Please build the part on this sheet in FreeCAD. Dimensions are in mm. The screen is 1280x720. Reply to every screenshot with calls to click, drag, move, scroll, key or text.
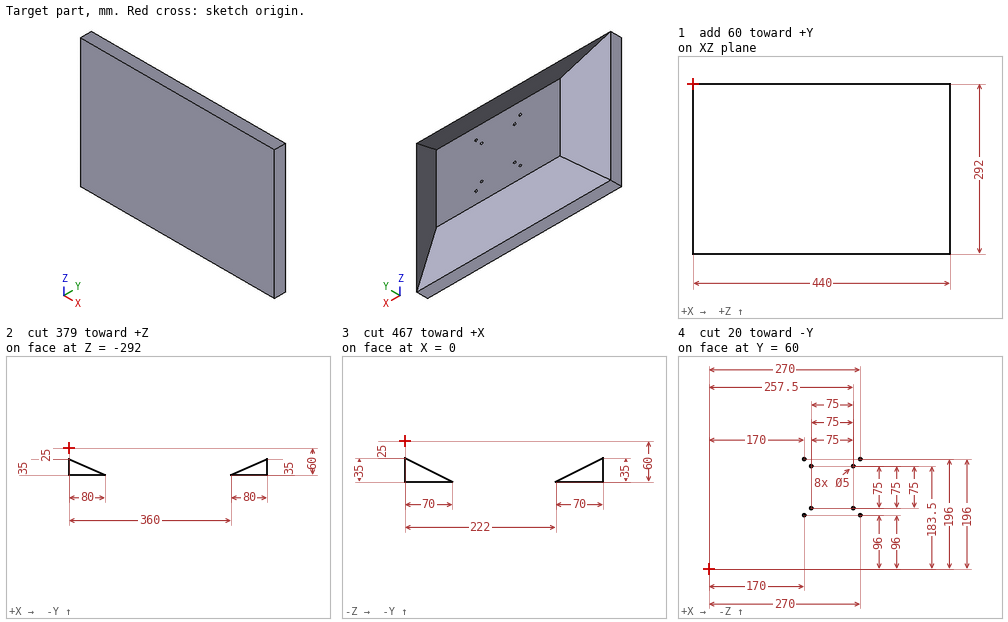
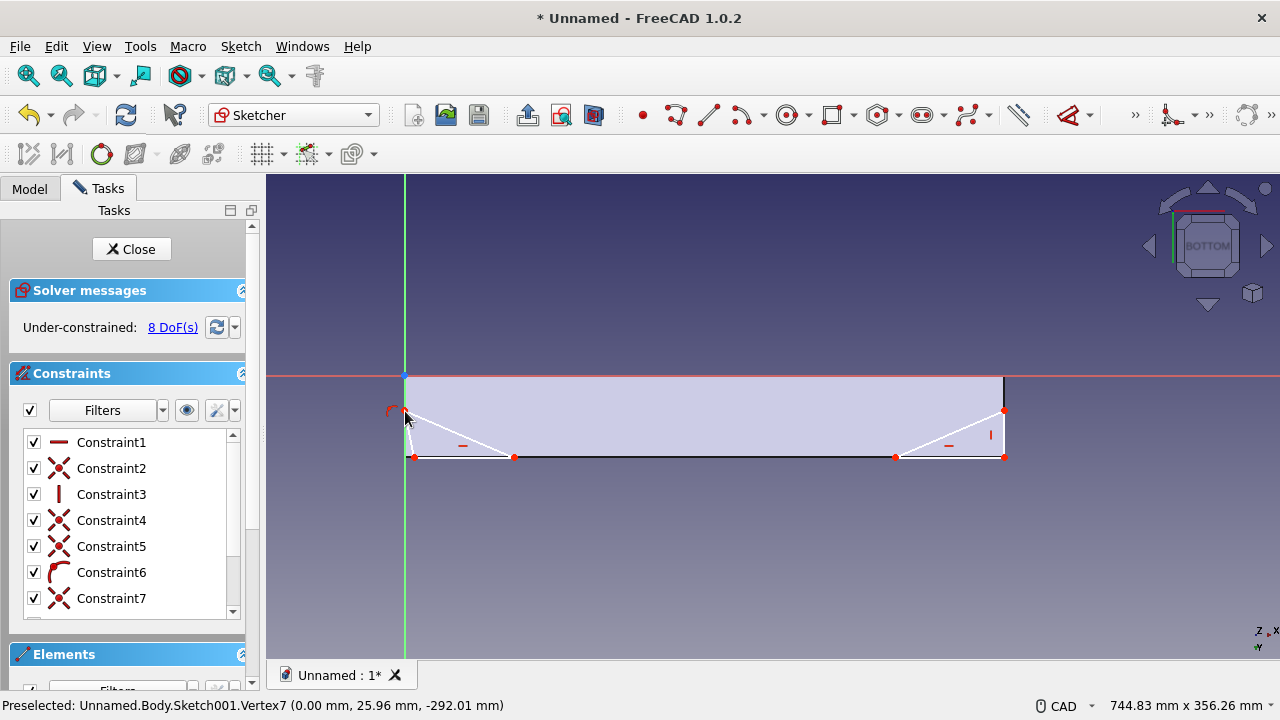
click(408, 425)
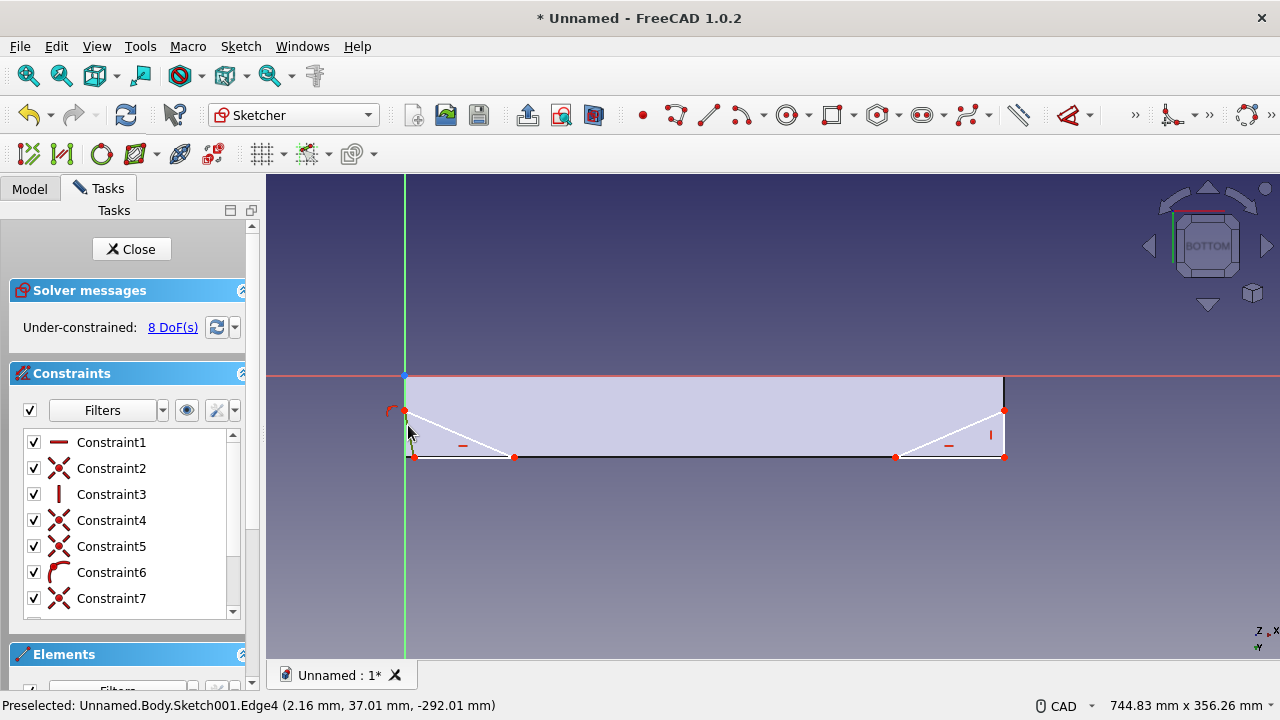
key(v)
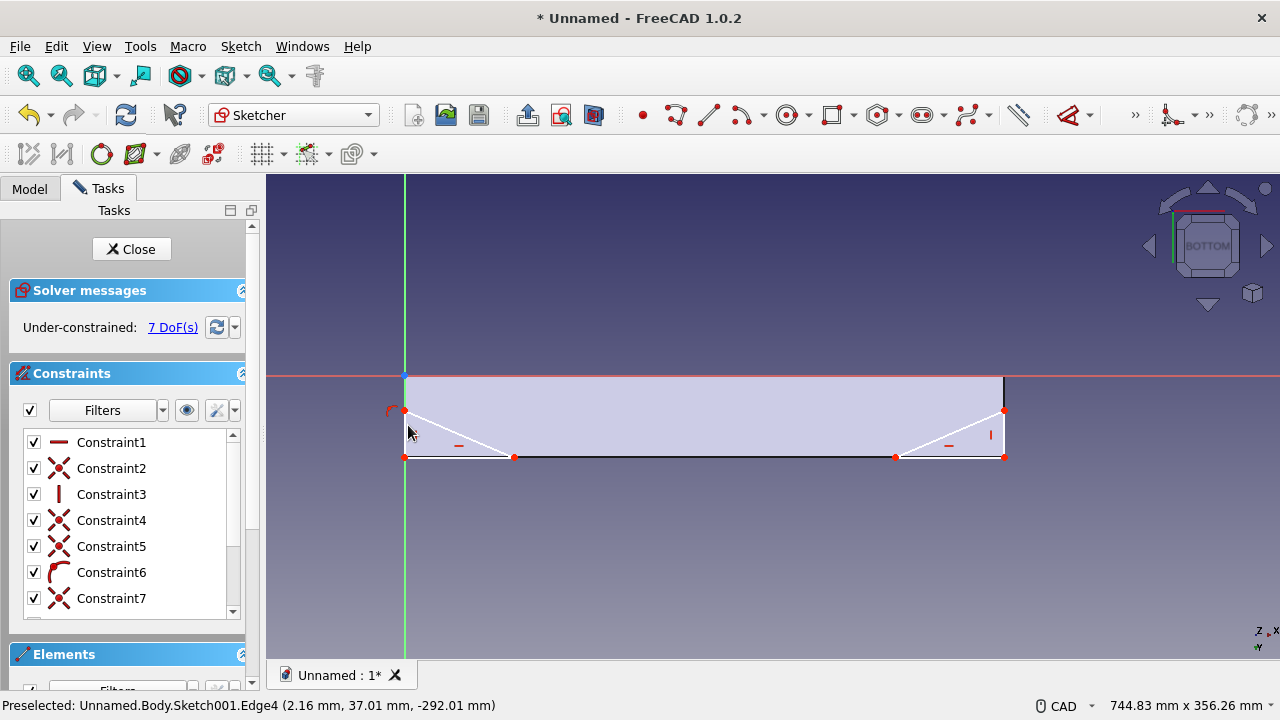
click(928, 458)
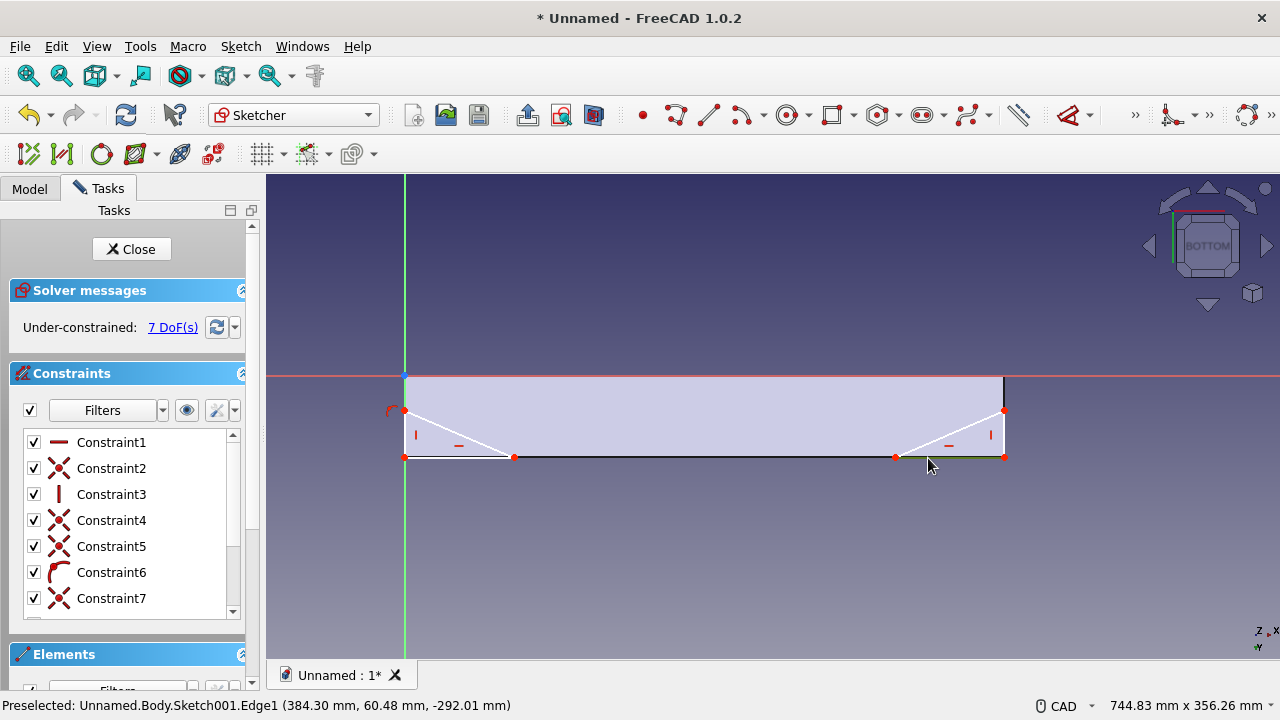
key(l)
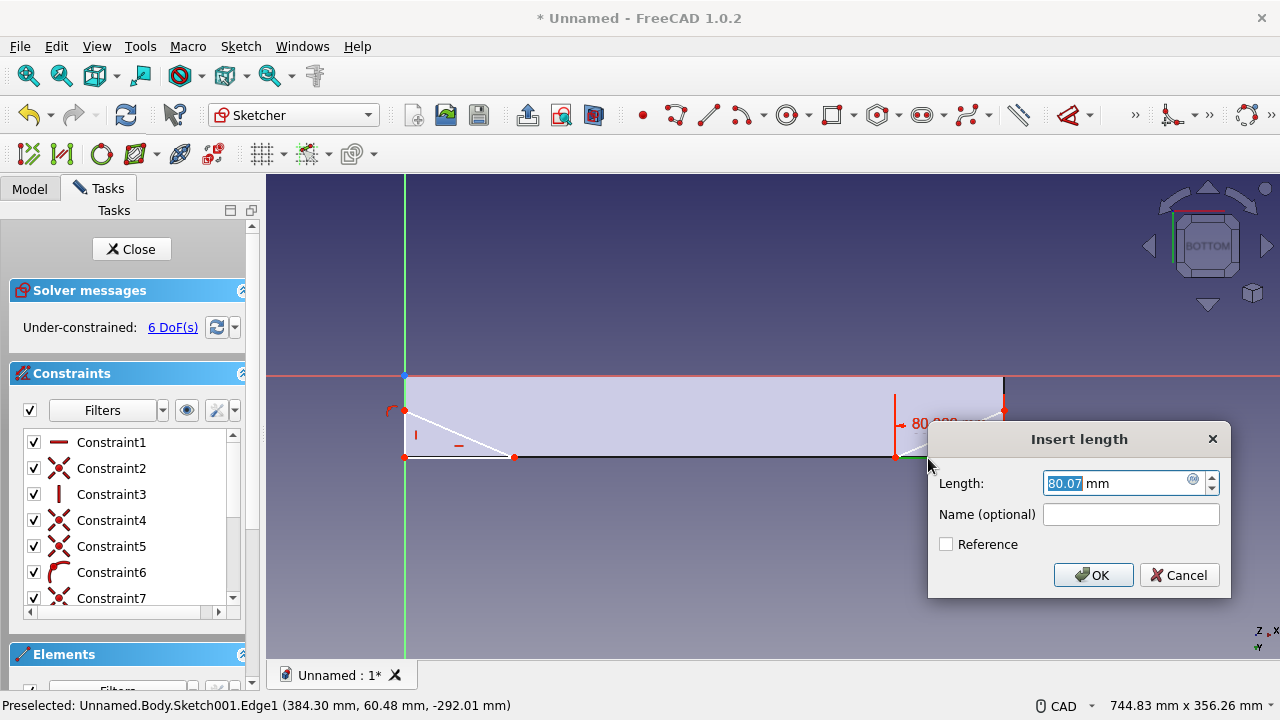
text(80)
key(Return)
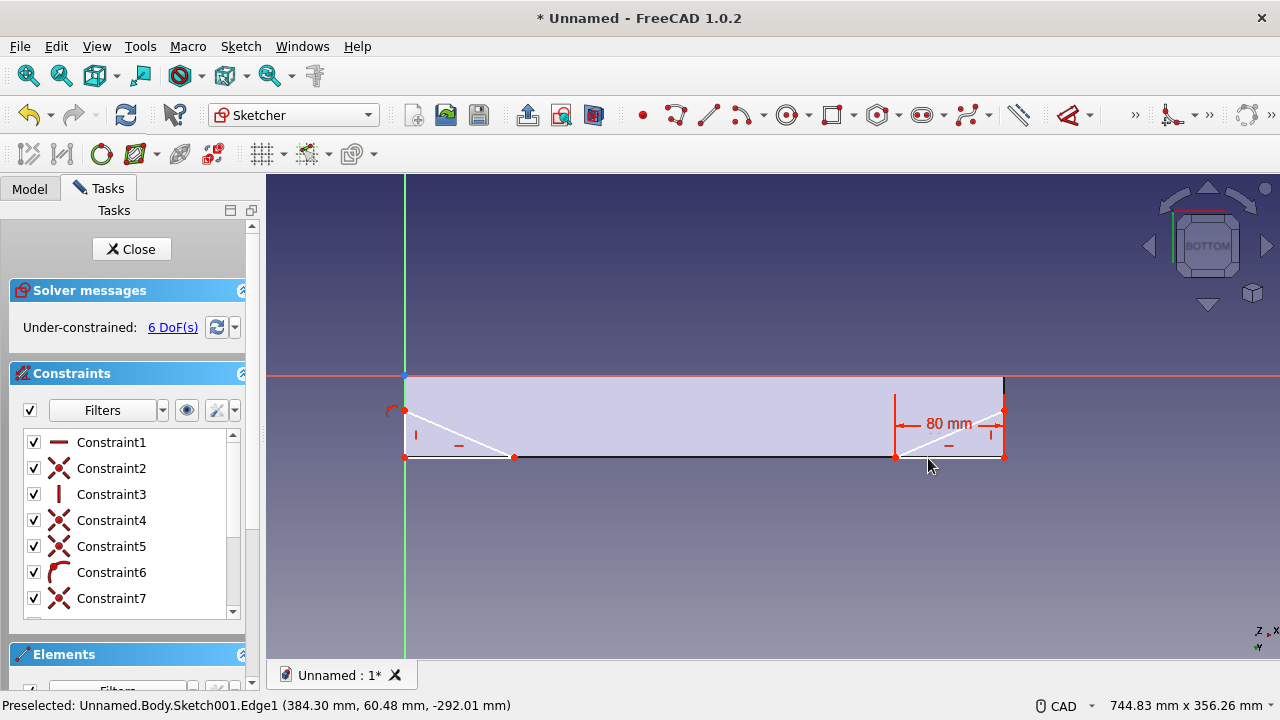
click(1004, 444)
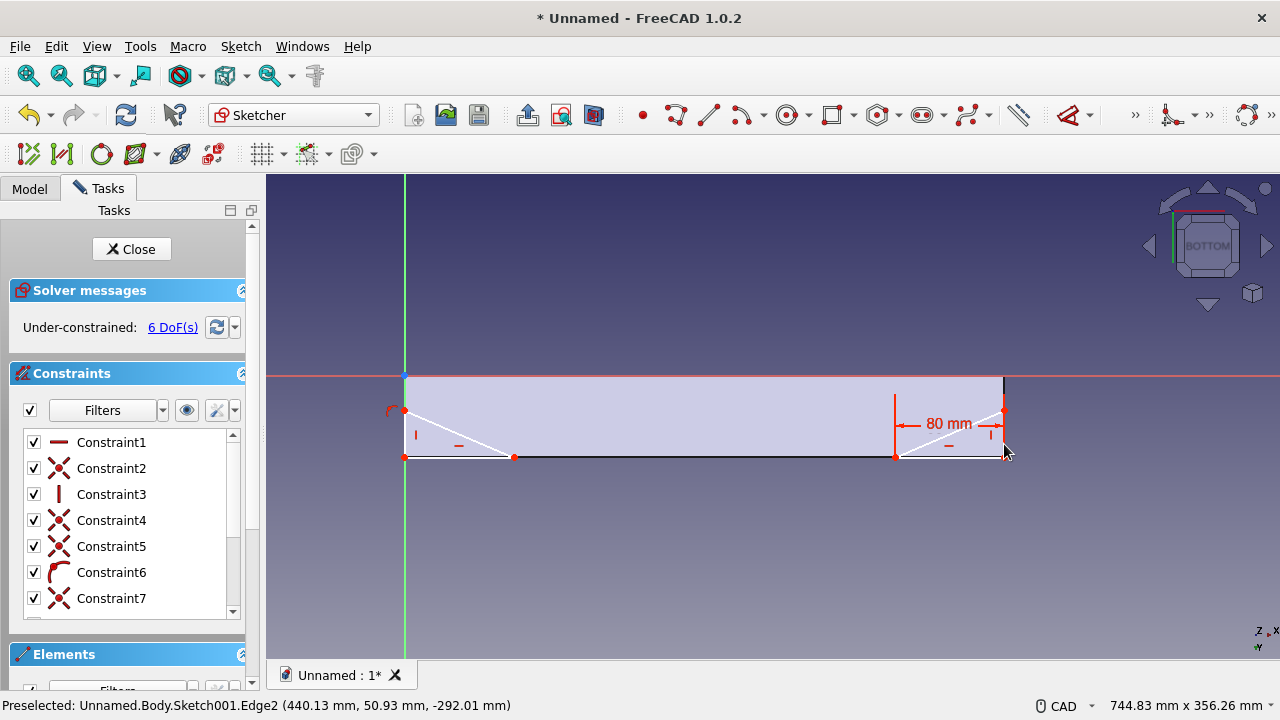
key(i)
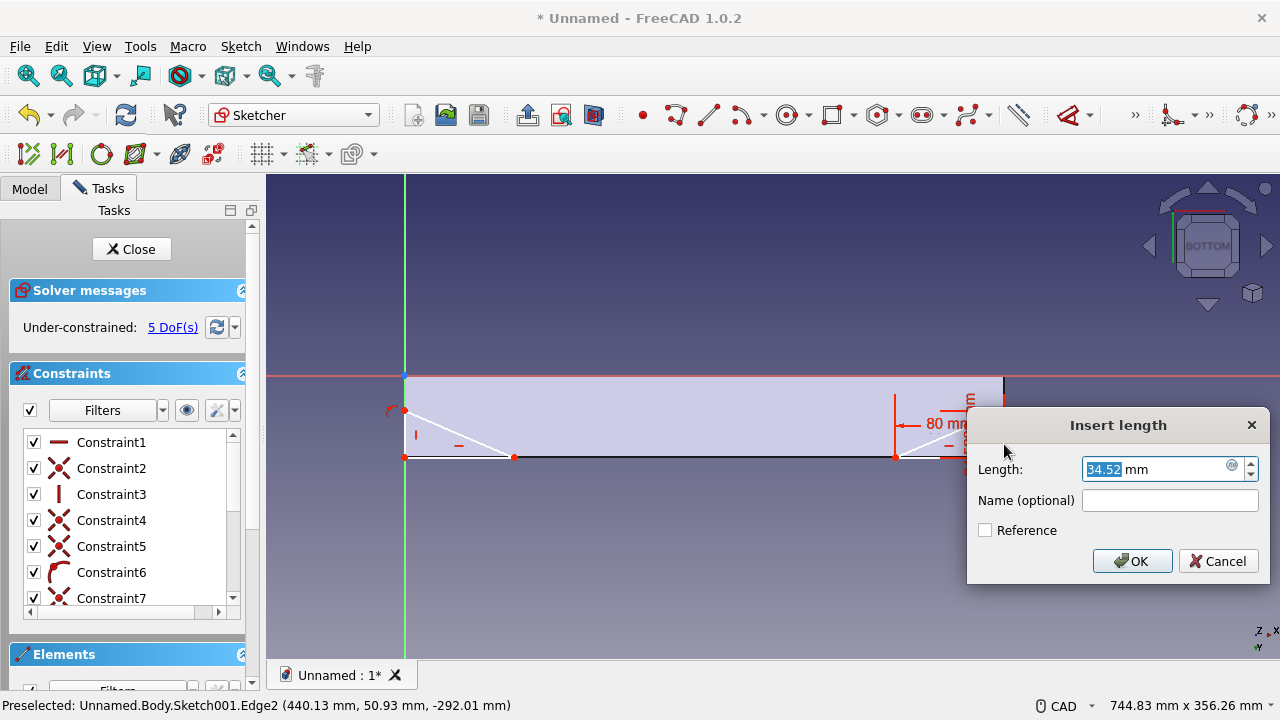
text(35)
key(Return)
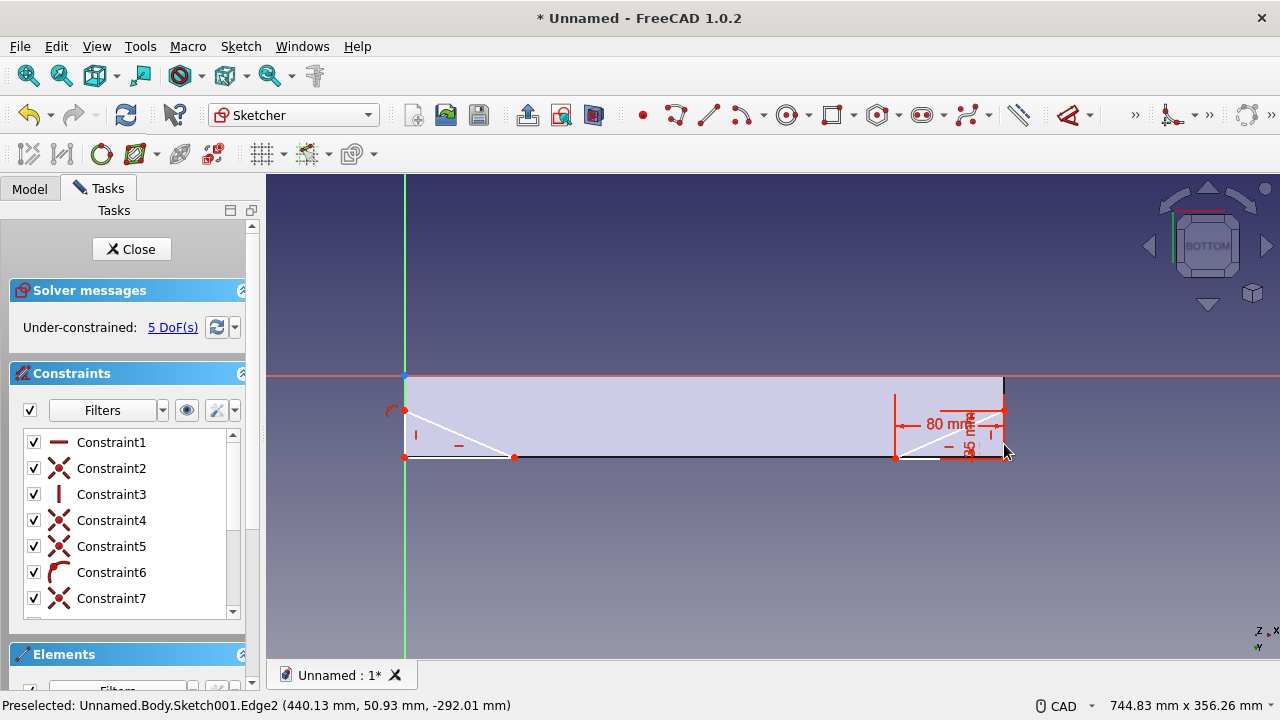
click(405, 425)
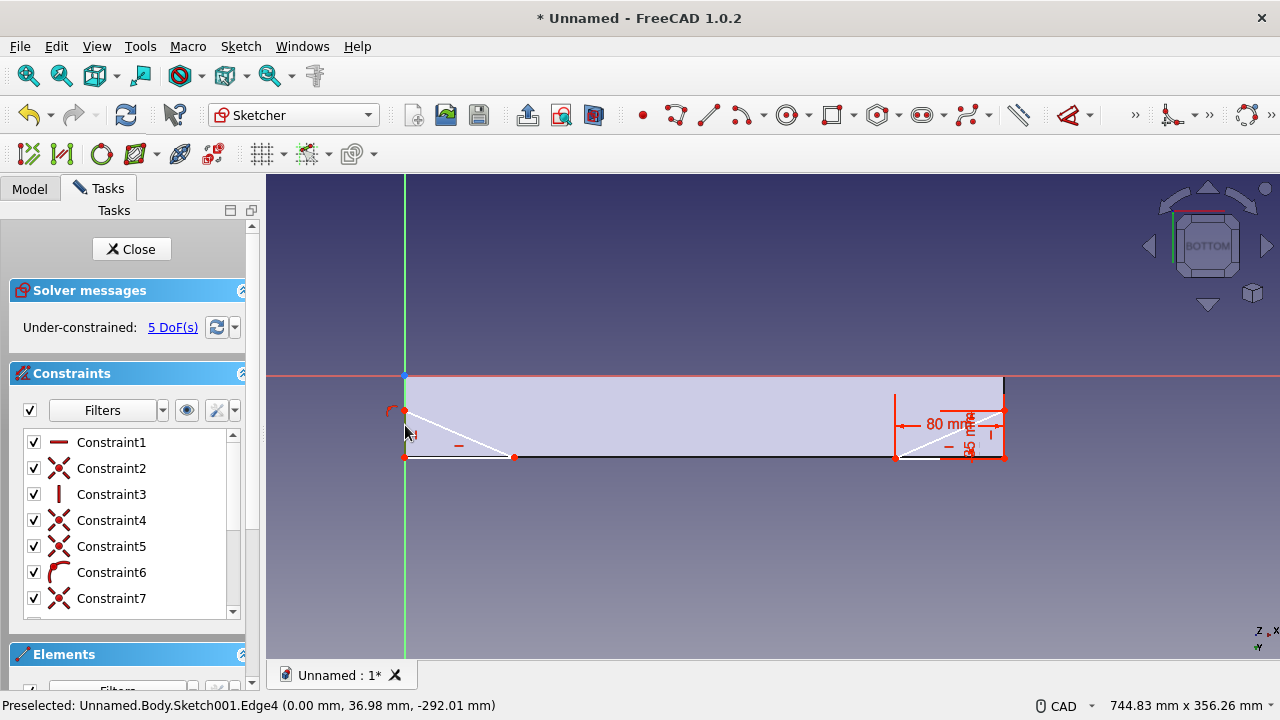
key(i)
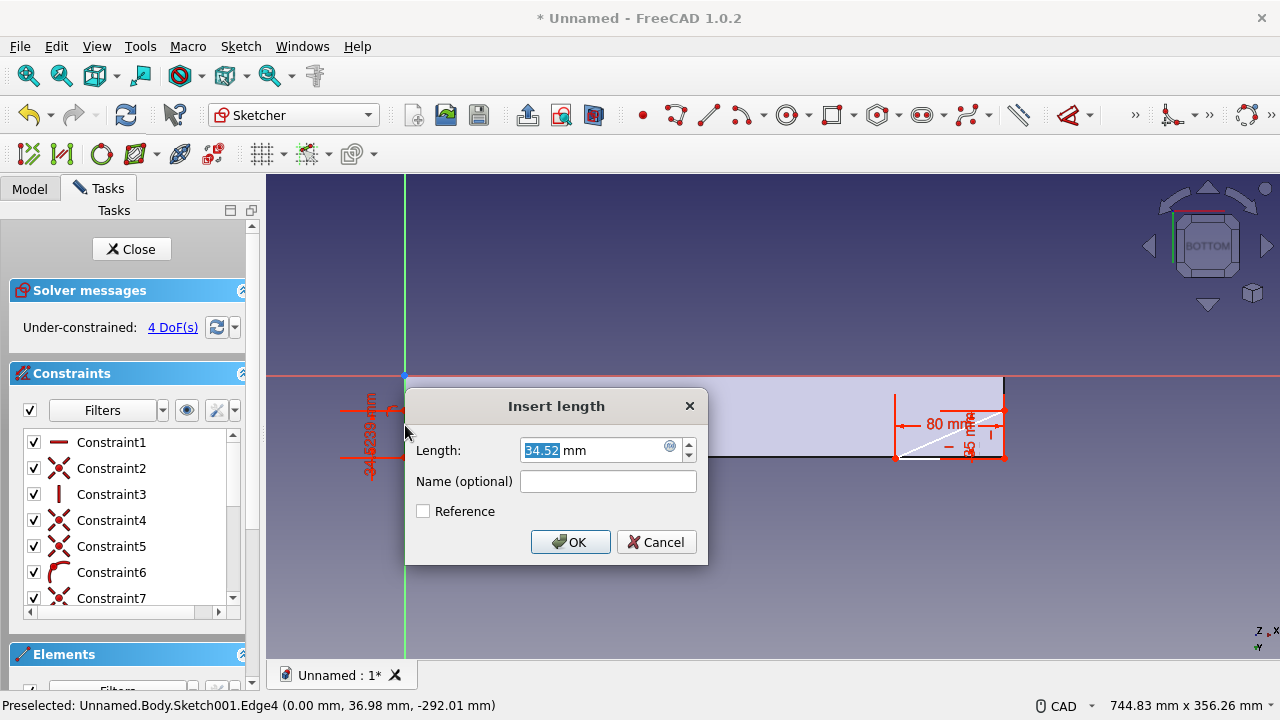
text(35)
key(Return)